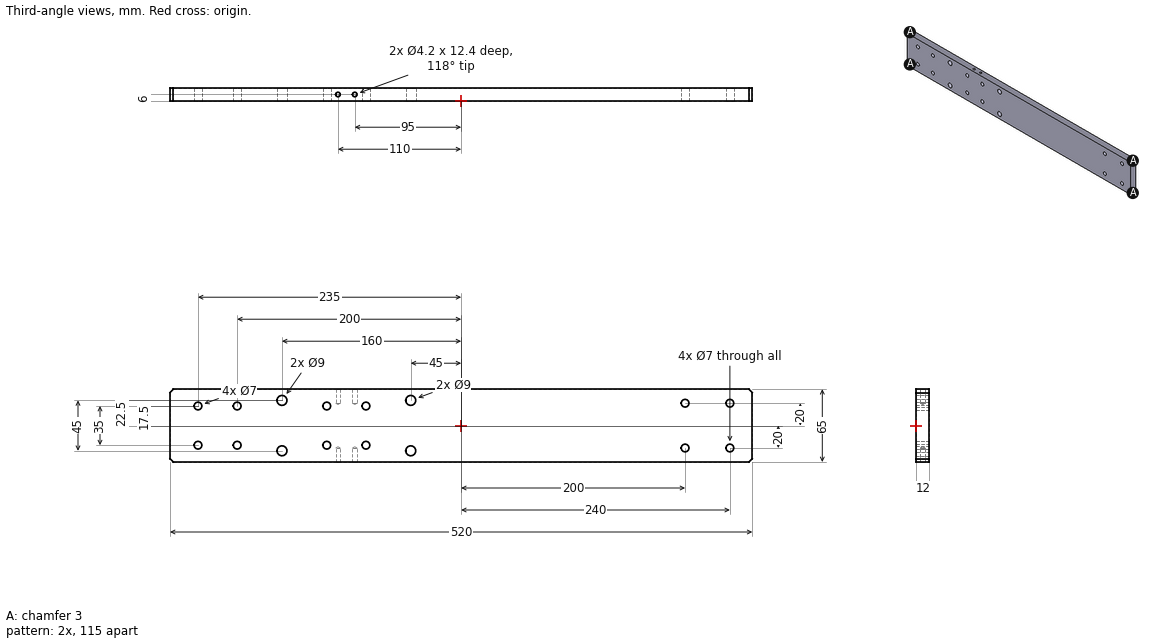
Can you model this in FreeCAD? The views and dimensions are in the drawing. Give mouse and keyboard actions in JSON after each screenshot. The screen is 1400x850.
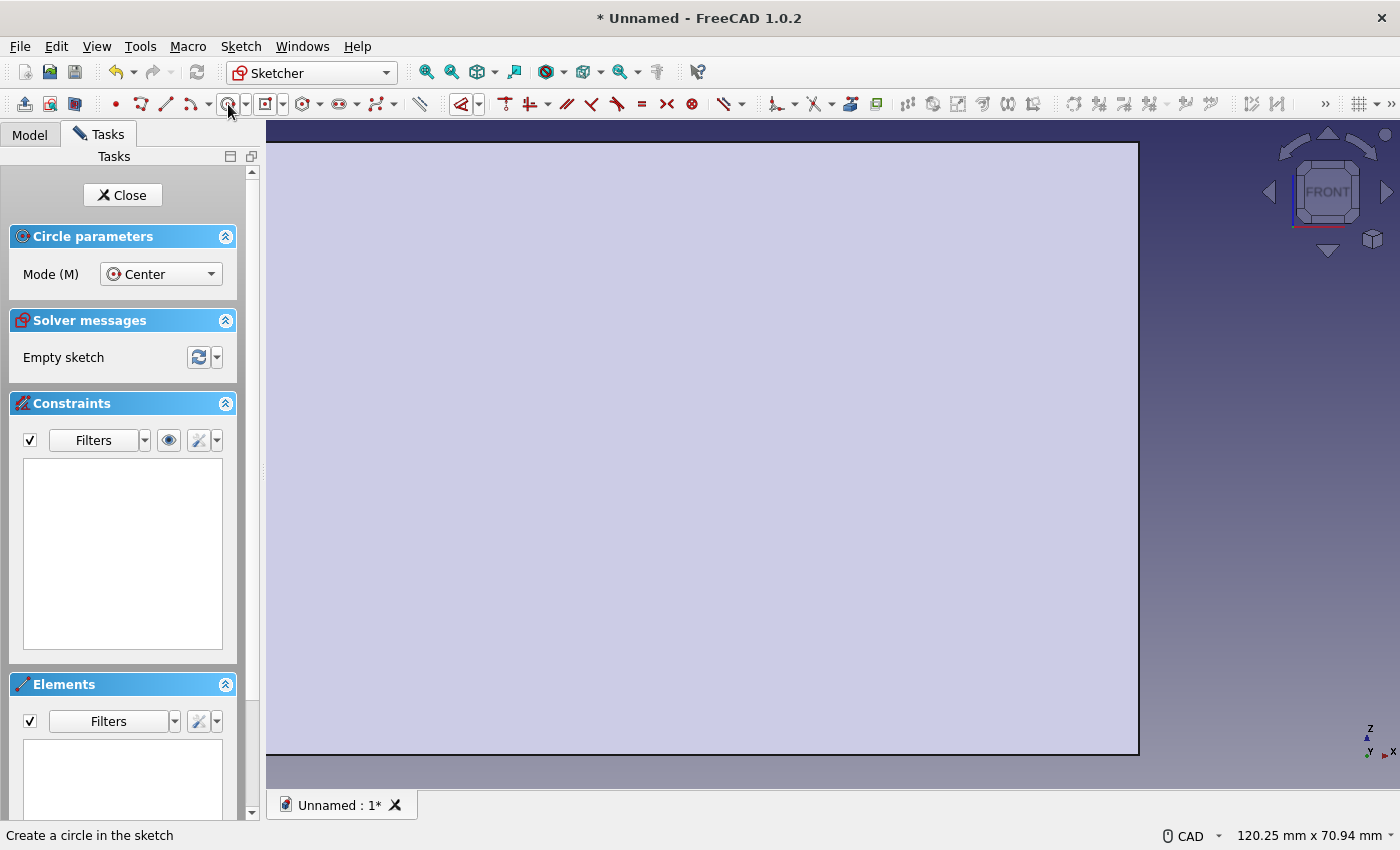
{"action": "left_click", "coordinate": [951, 637]}
{"action": "left_click", "coordinate": [974, 613]}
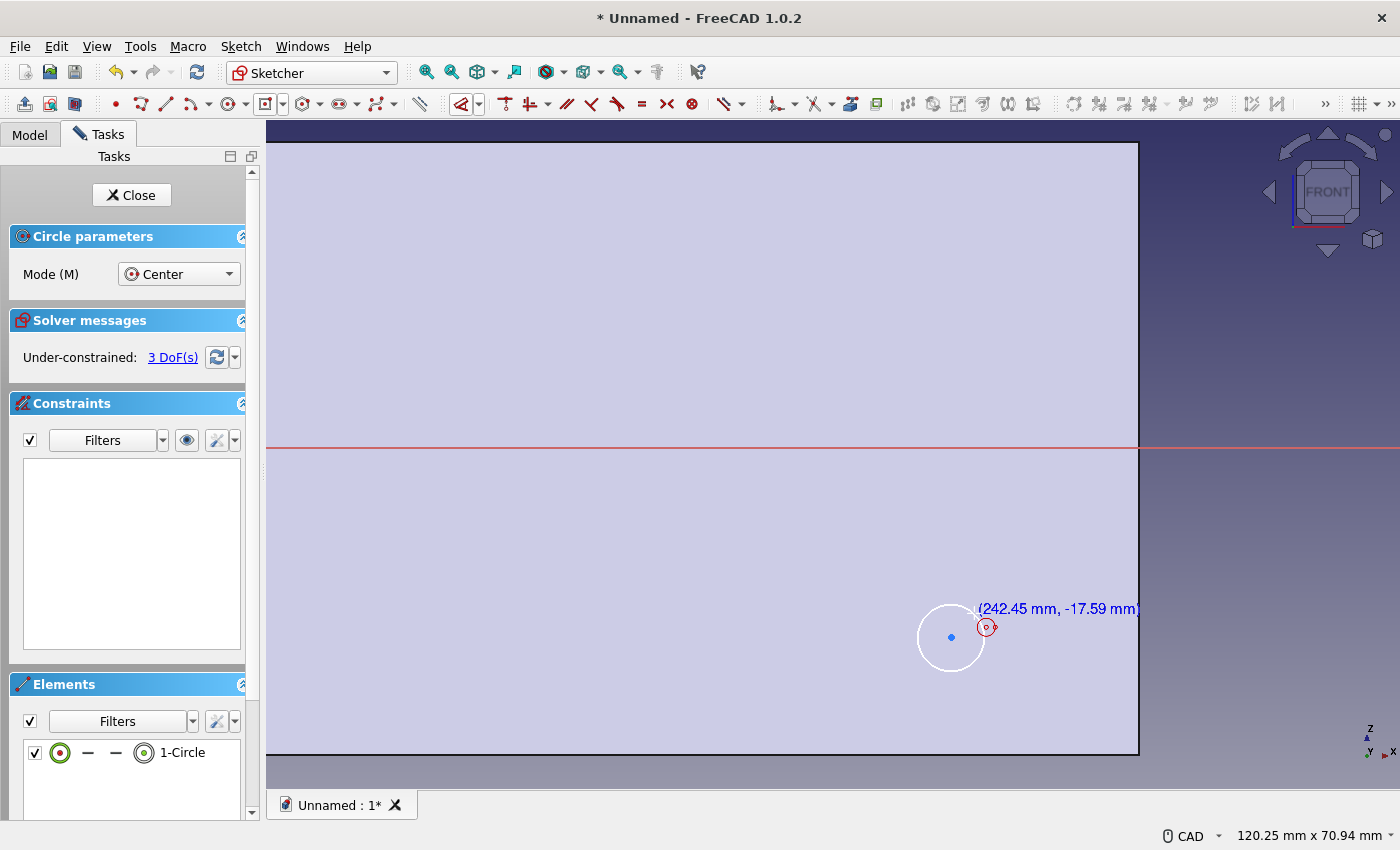
{"action": "left_click", "coordinate": [574, 637]}
{"action": "left_click", "coordinate": [597, 613]}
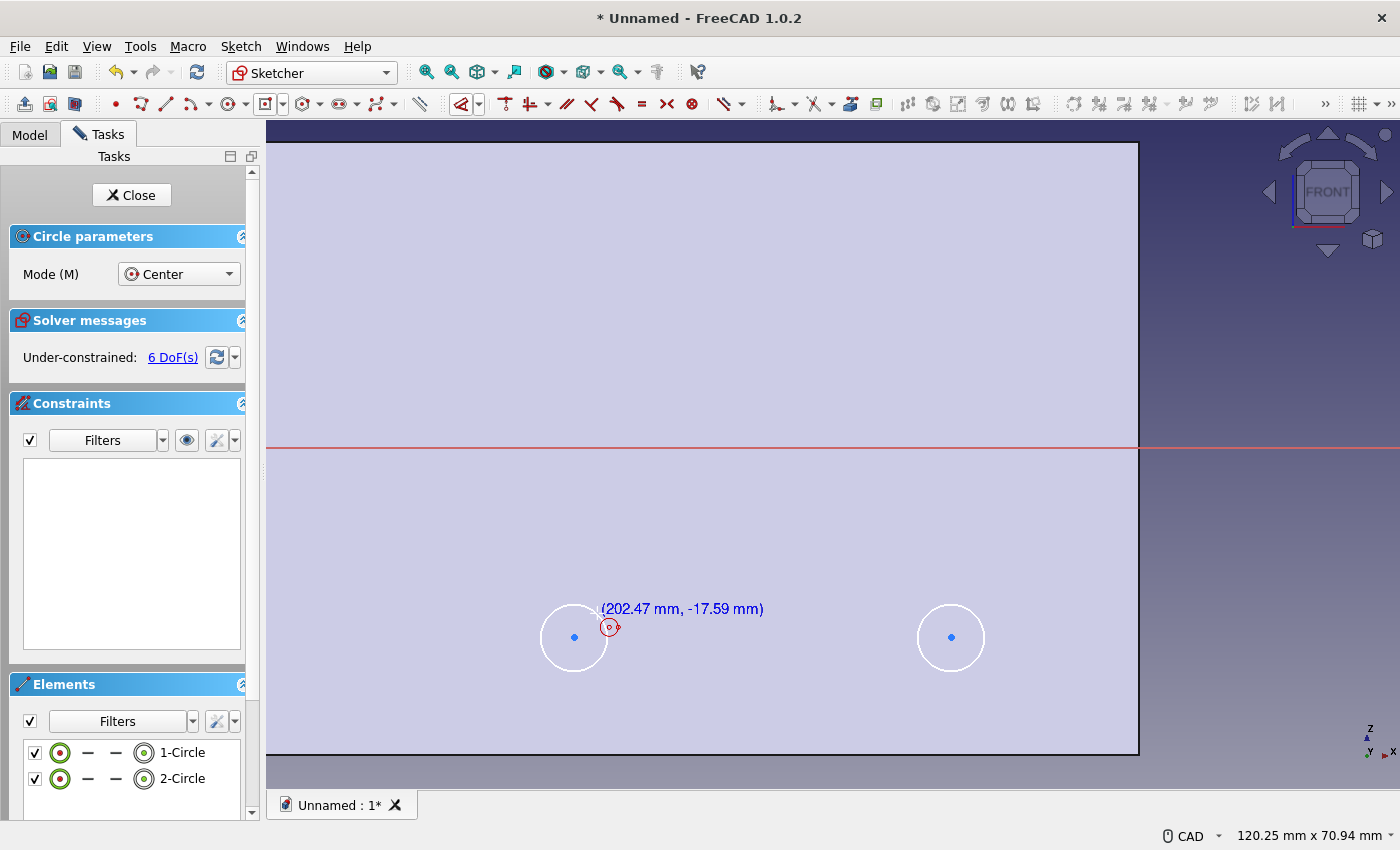
{"action": "left_click", "coordinate": [574, 259]}
{"action": "left_click", "coordinate": [597, 236]}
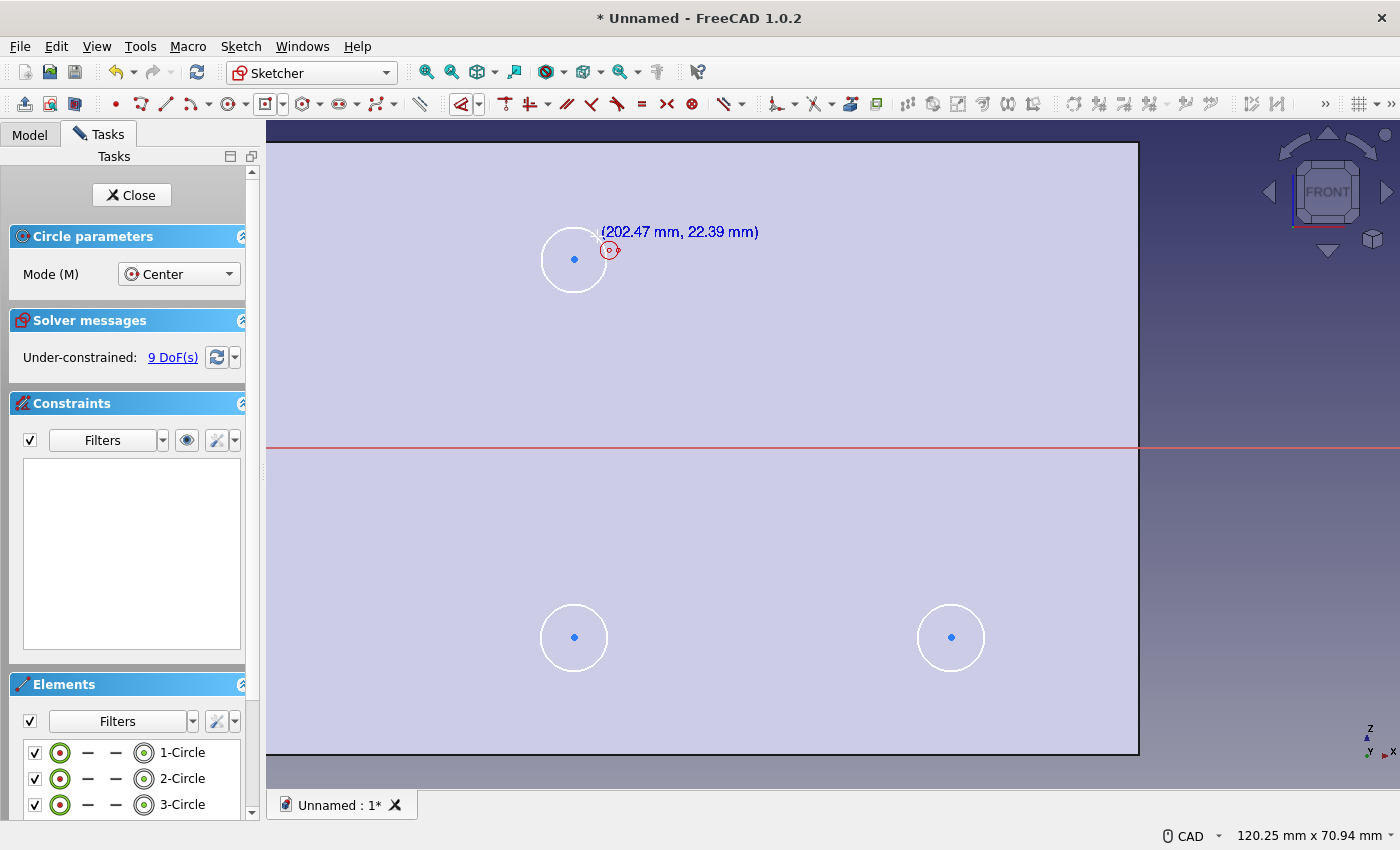
{"action": "left_click", "coordinate": [951, 259]}
{"action": "left_click", "coordinate": [974, 236]}
{"action": "key", "text": "Escape"}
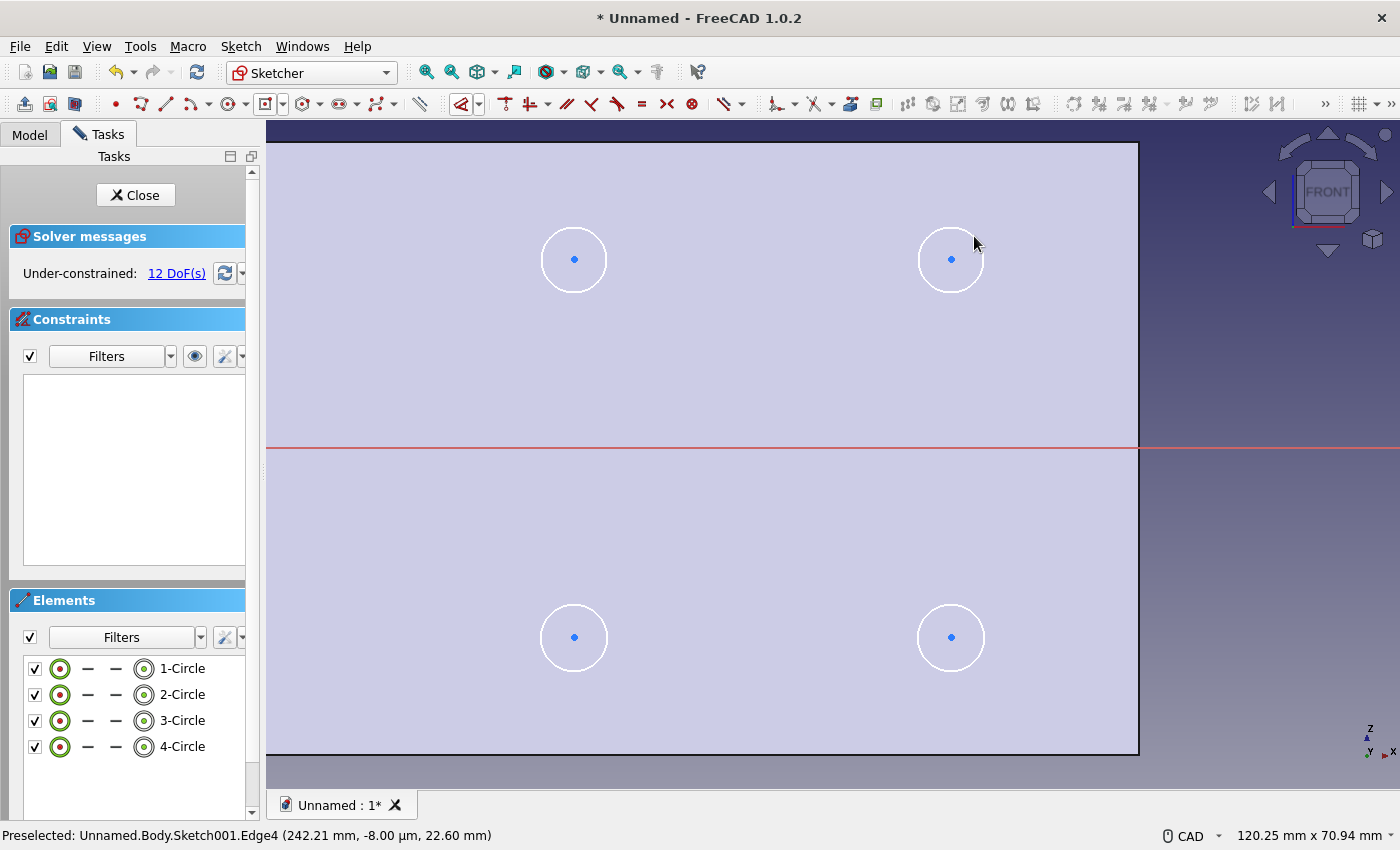
{"action": "left_click", "coordinate": [974, 614]}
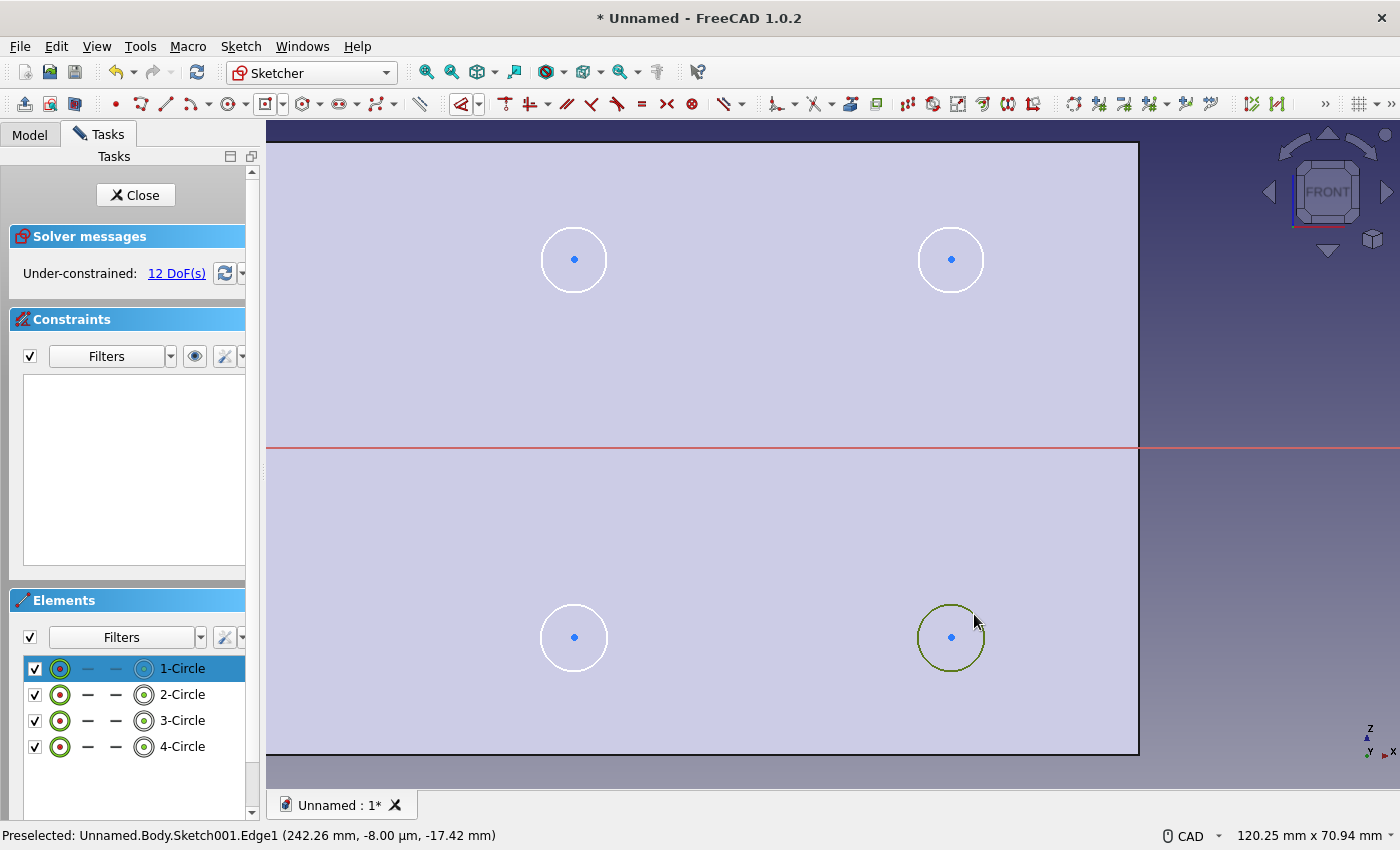
{"action": "left_click", "coordinate": [597, 614]}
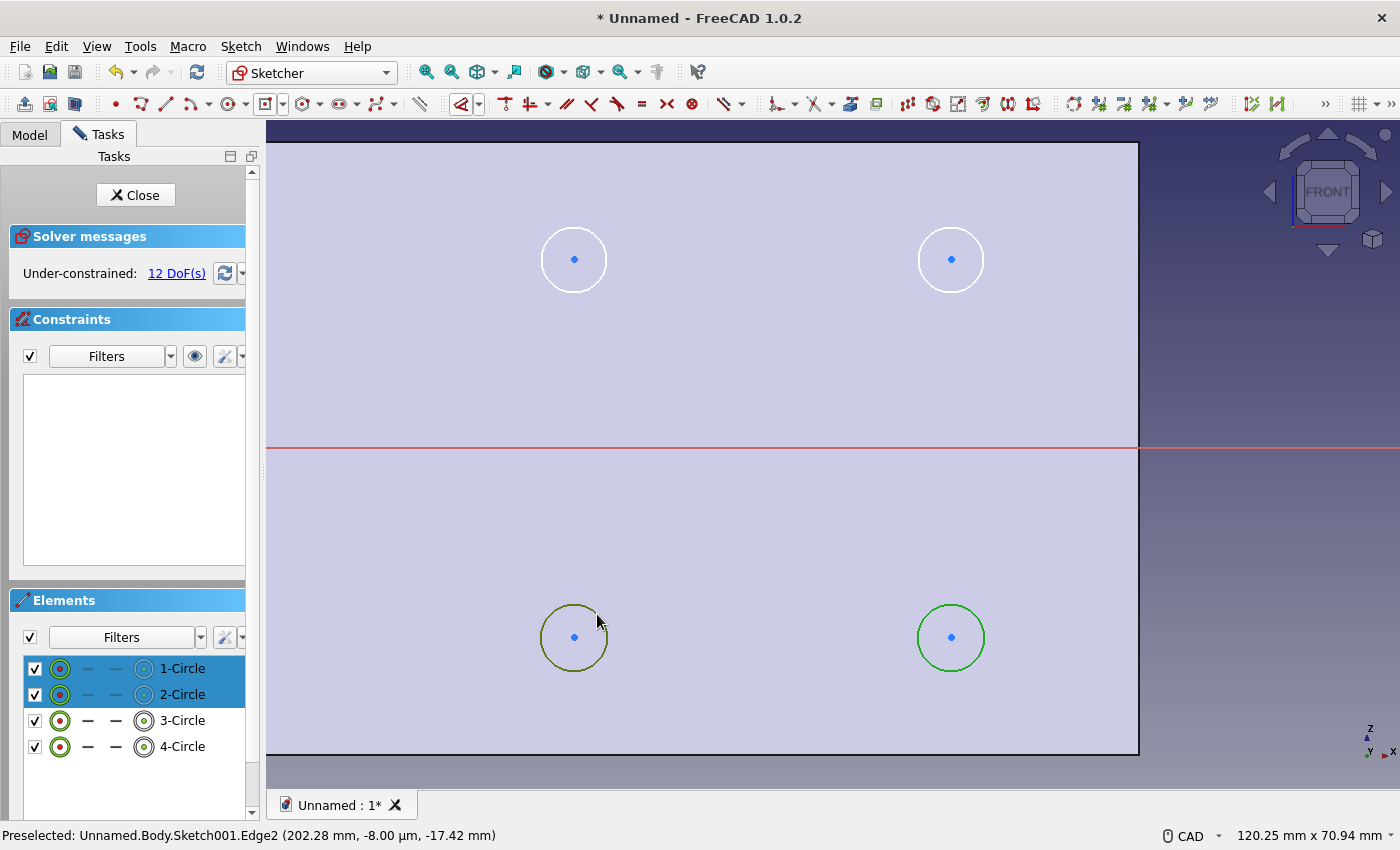
{"action": "left_click", "coordinate": [597, 237]}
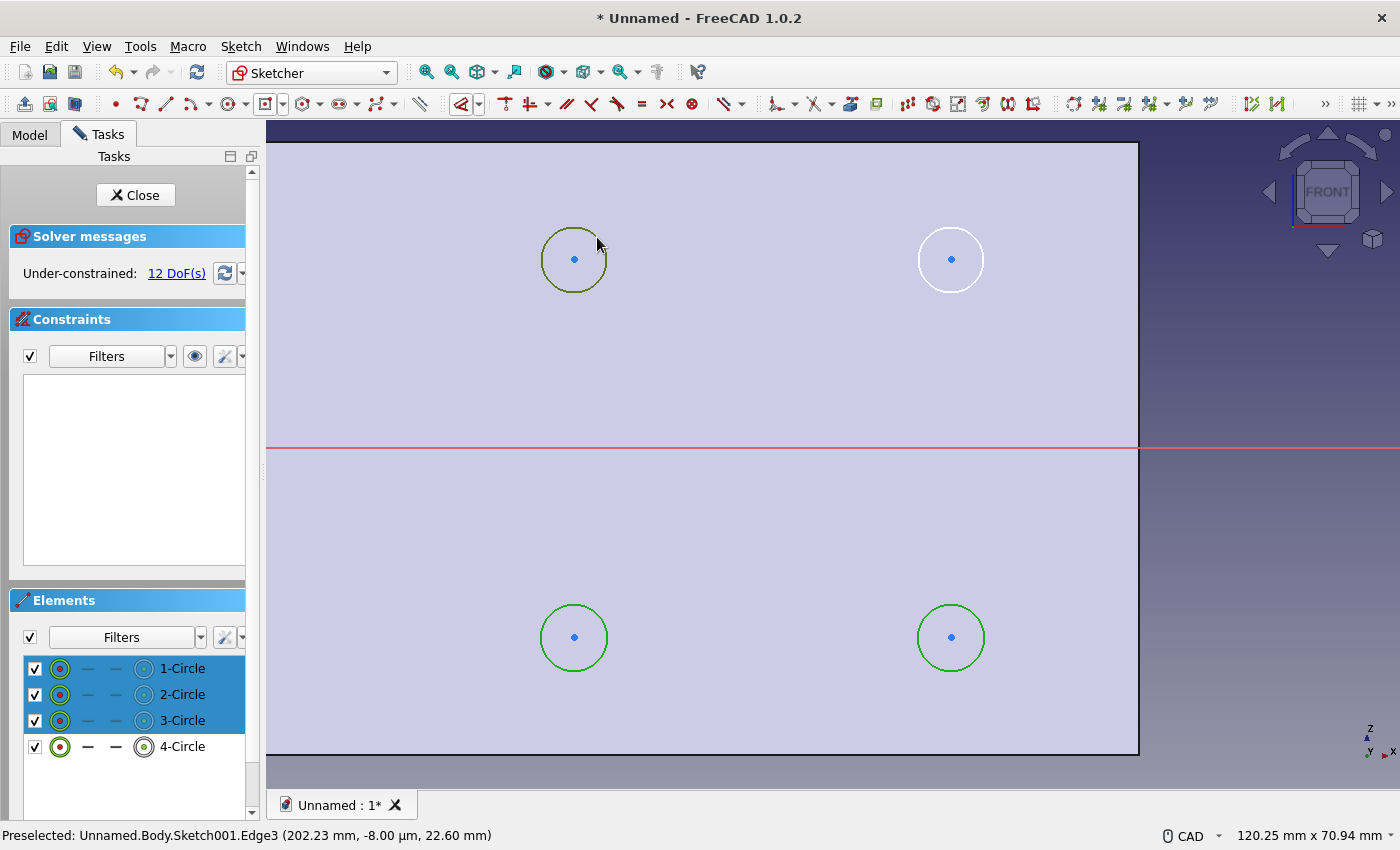
{"action": "left_click", "coordinate": [974, 237]}